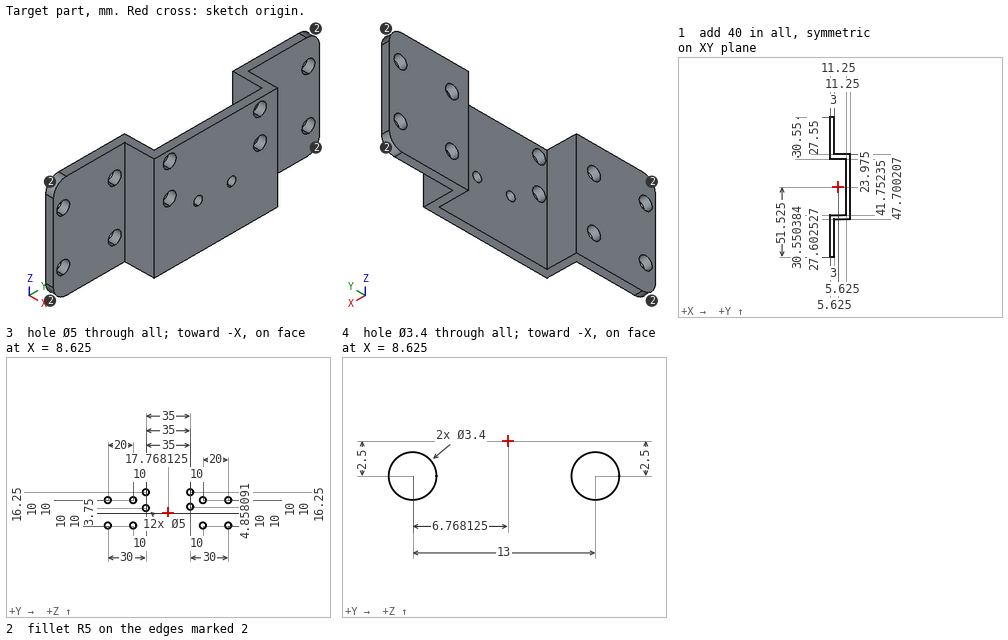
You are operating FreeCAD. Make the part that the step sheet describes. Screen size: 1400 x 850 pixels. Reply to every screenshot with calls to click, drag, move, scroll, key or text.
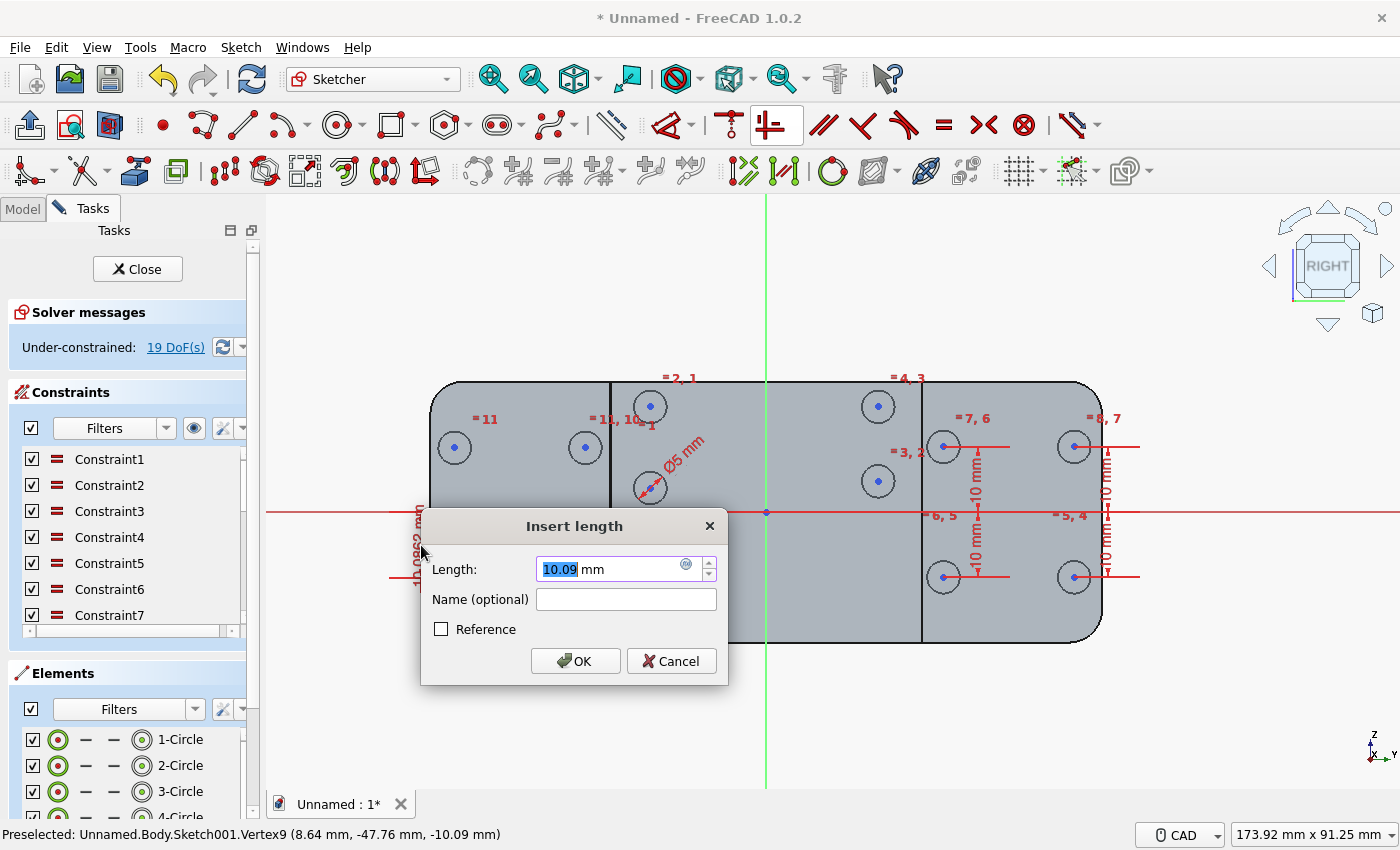
text(10)
key(Return)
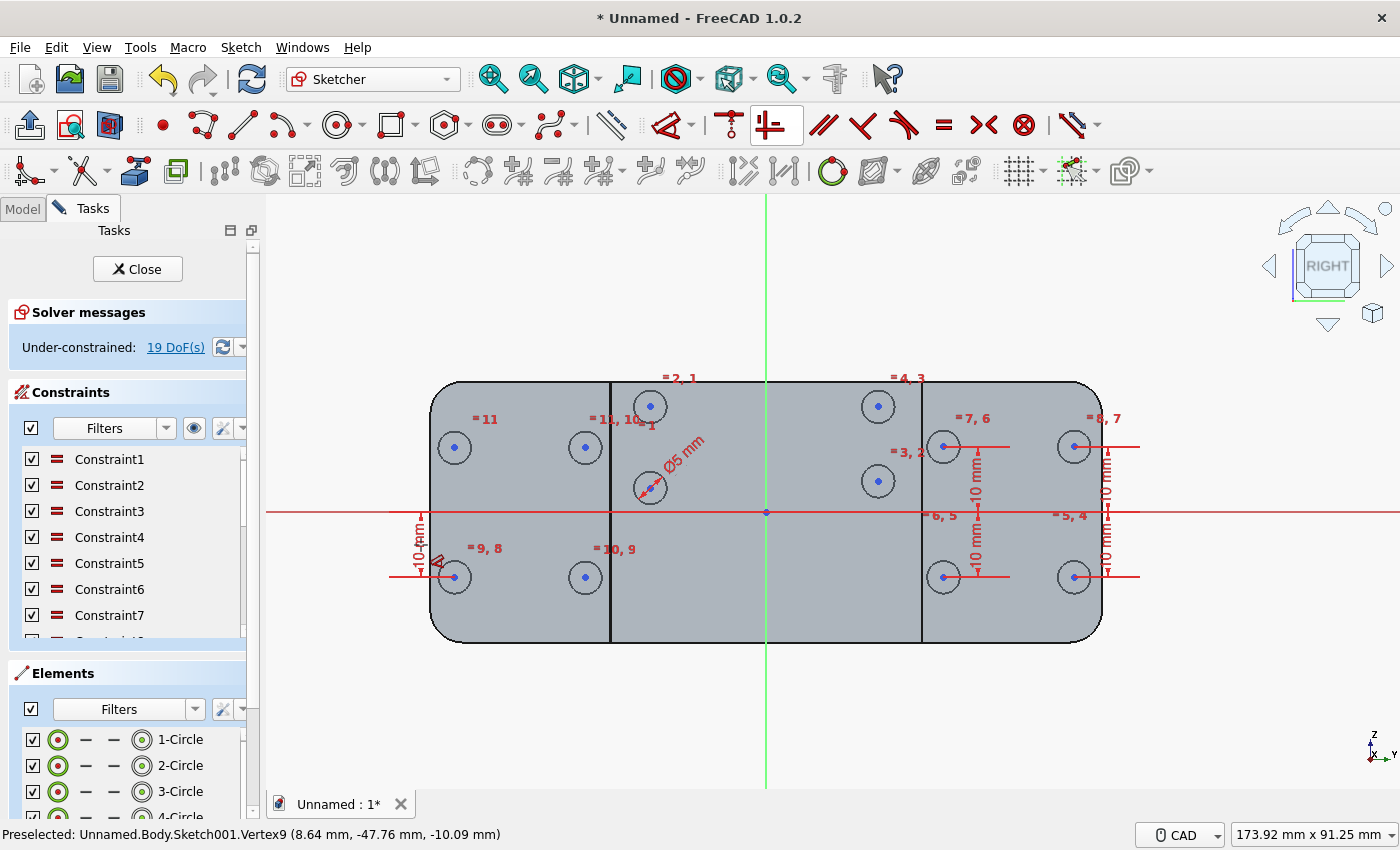
click(585, 578)
click(551, 545)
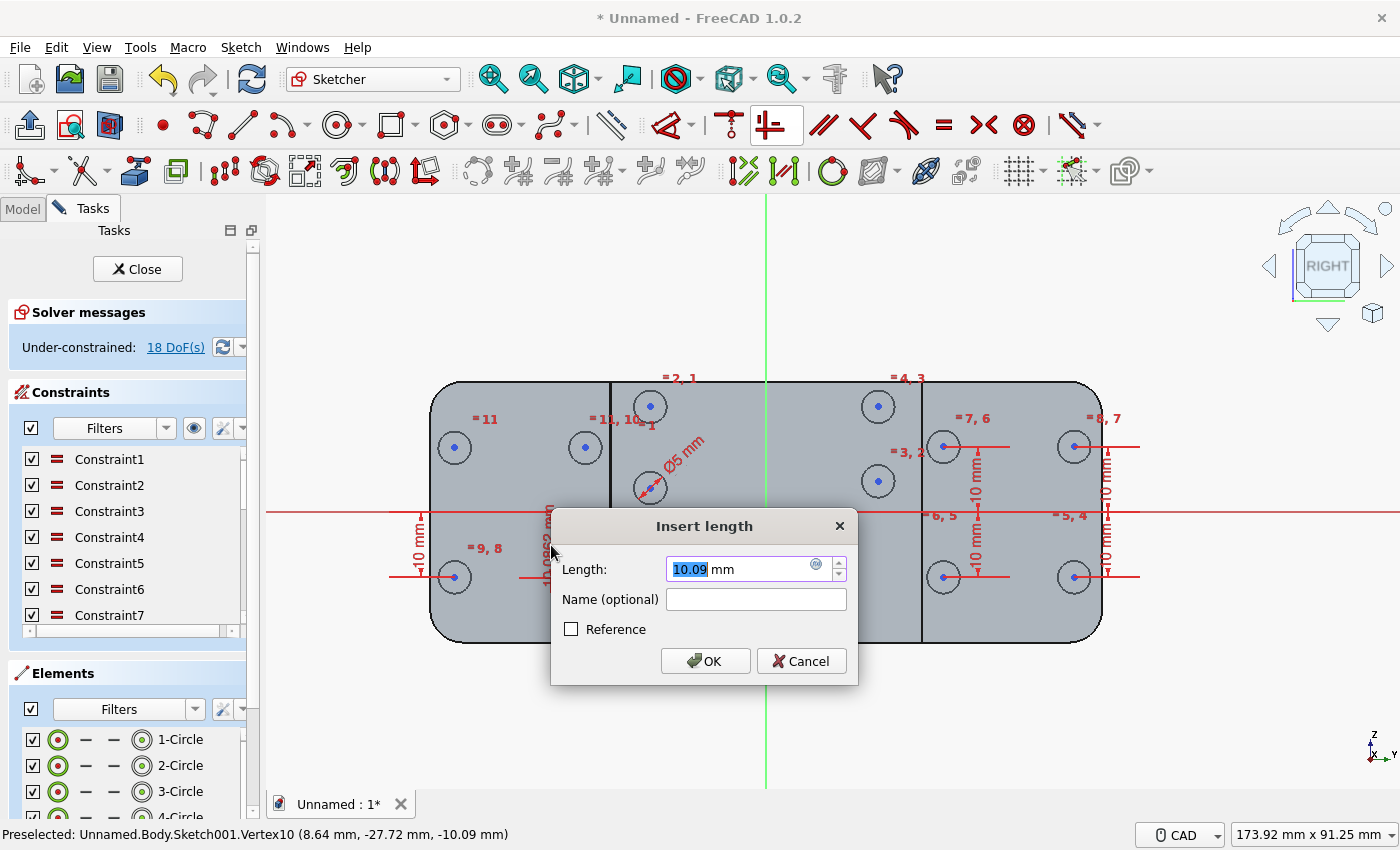
text(10)
key(Return)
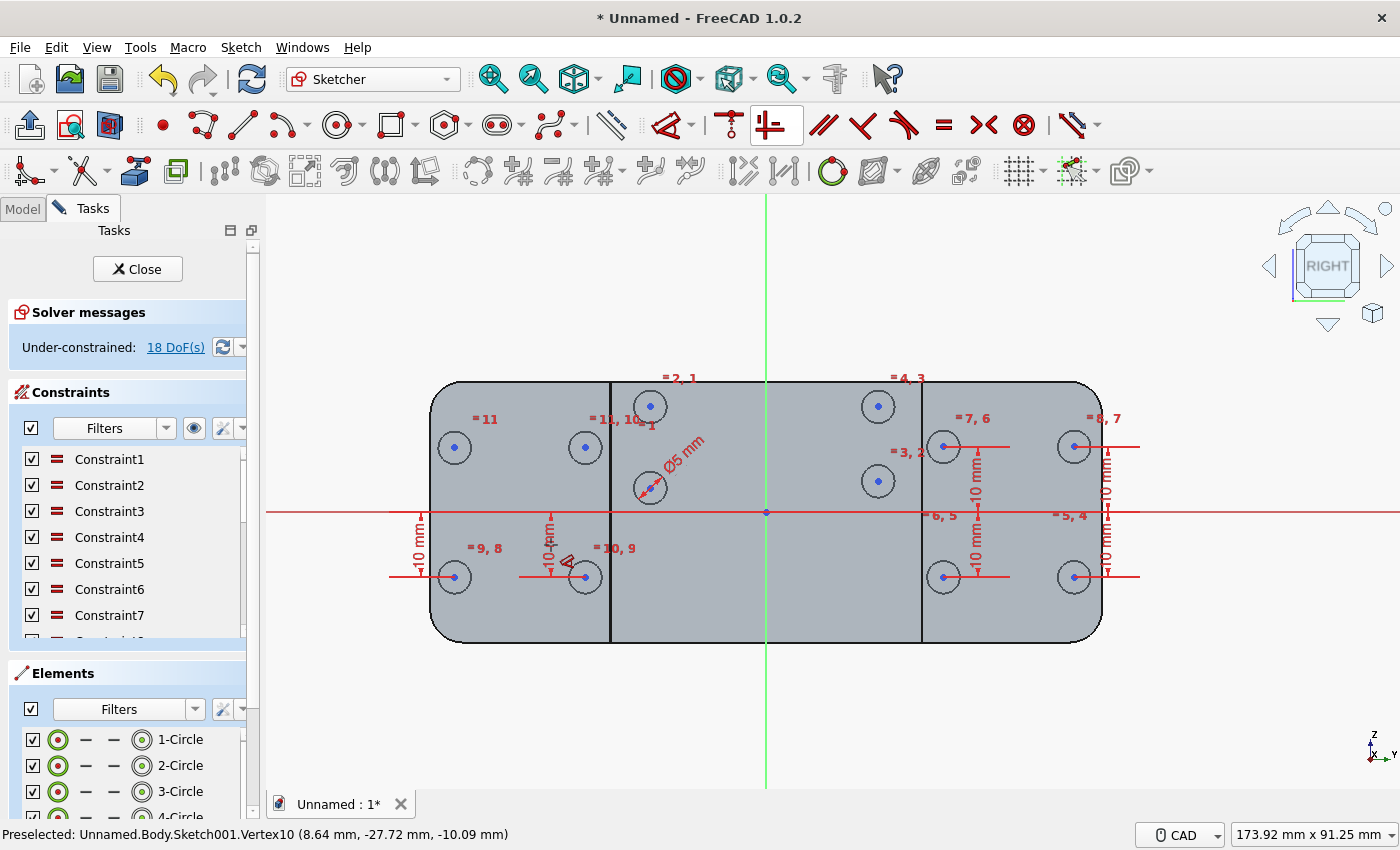
click(585, 448)
click(551, 480)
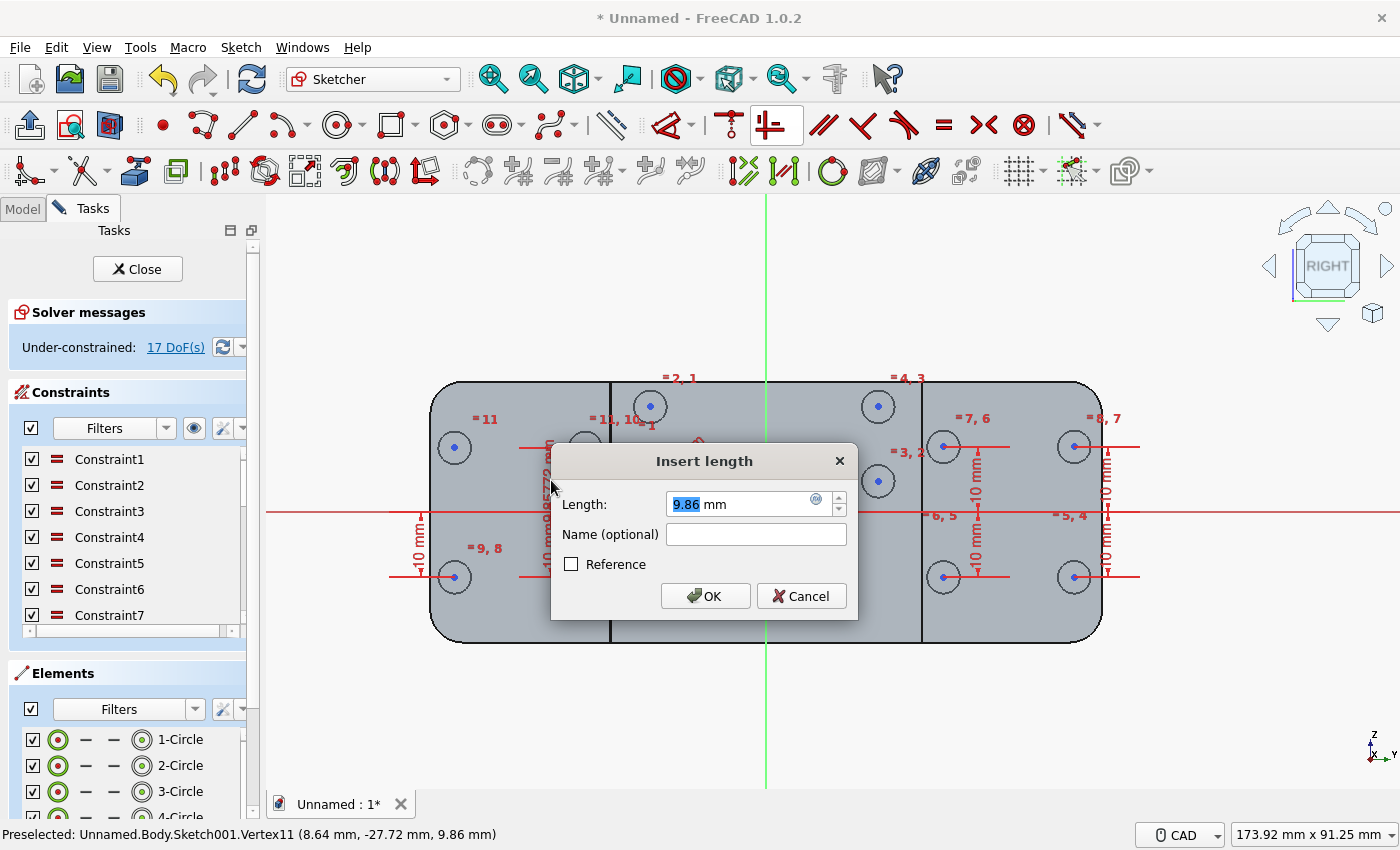
text(10)
key(Return)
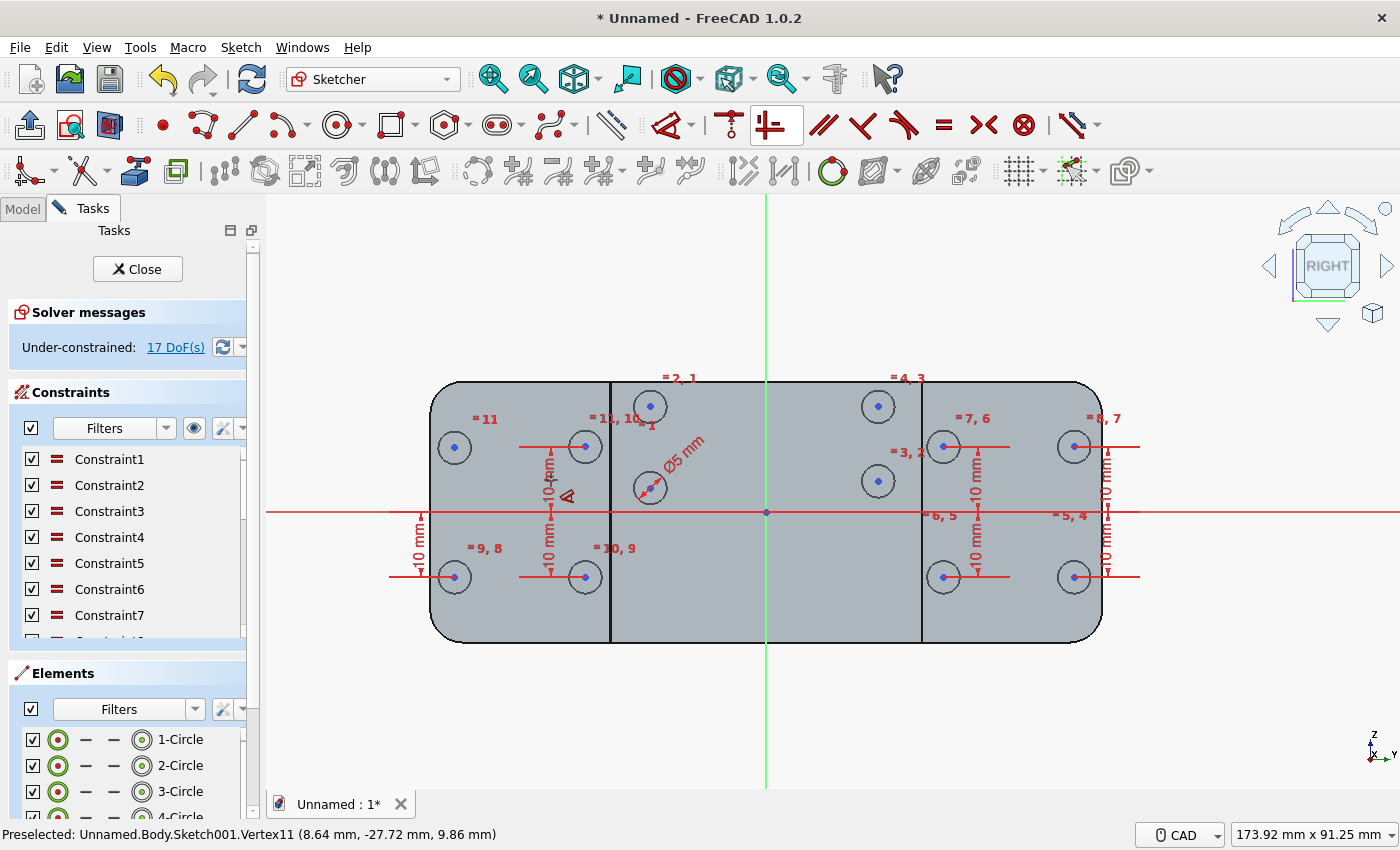
click(455, 448)
click(421, 480)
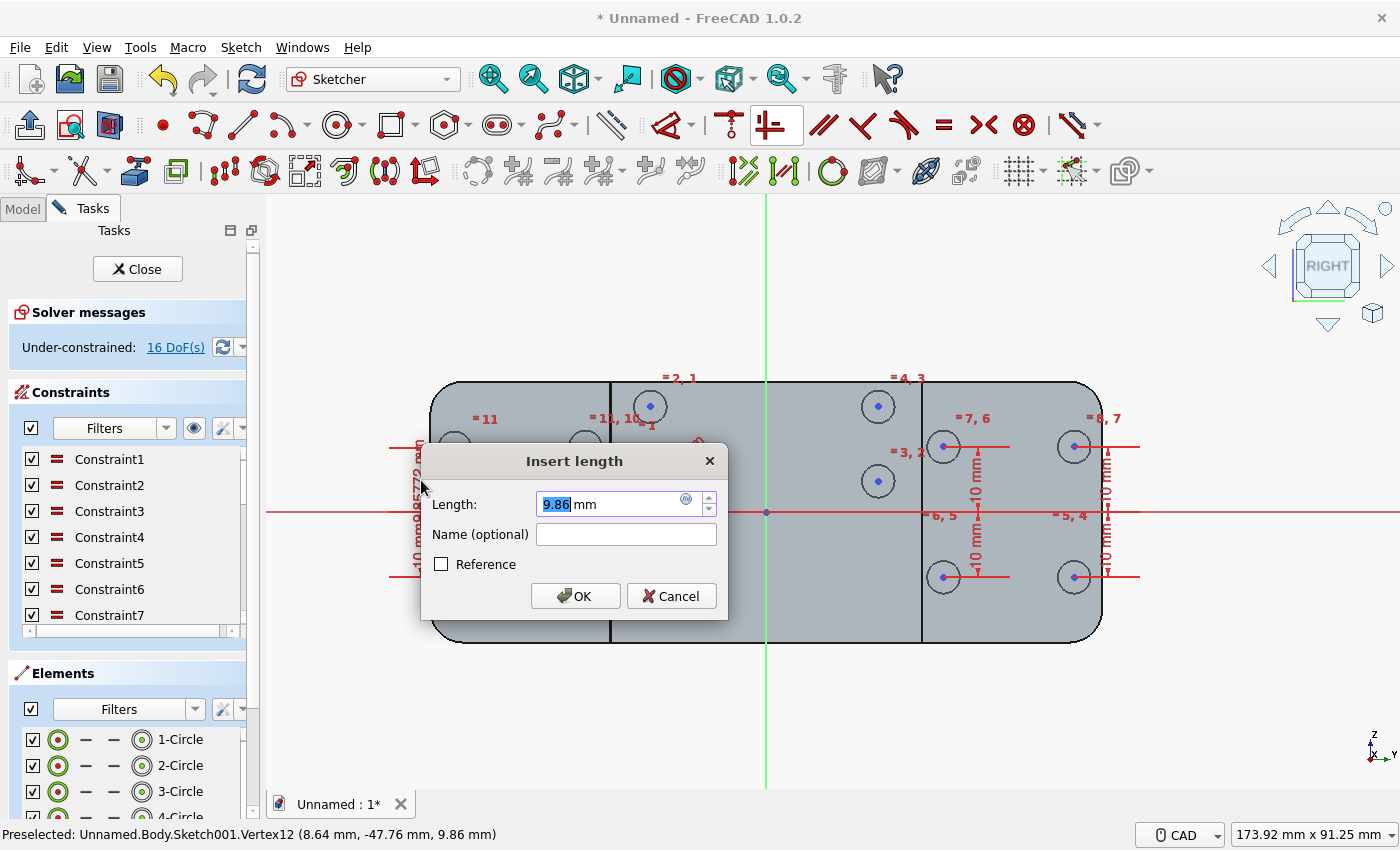
text(10)
key(Return)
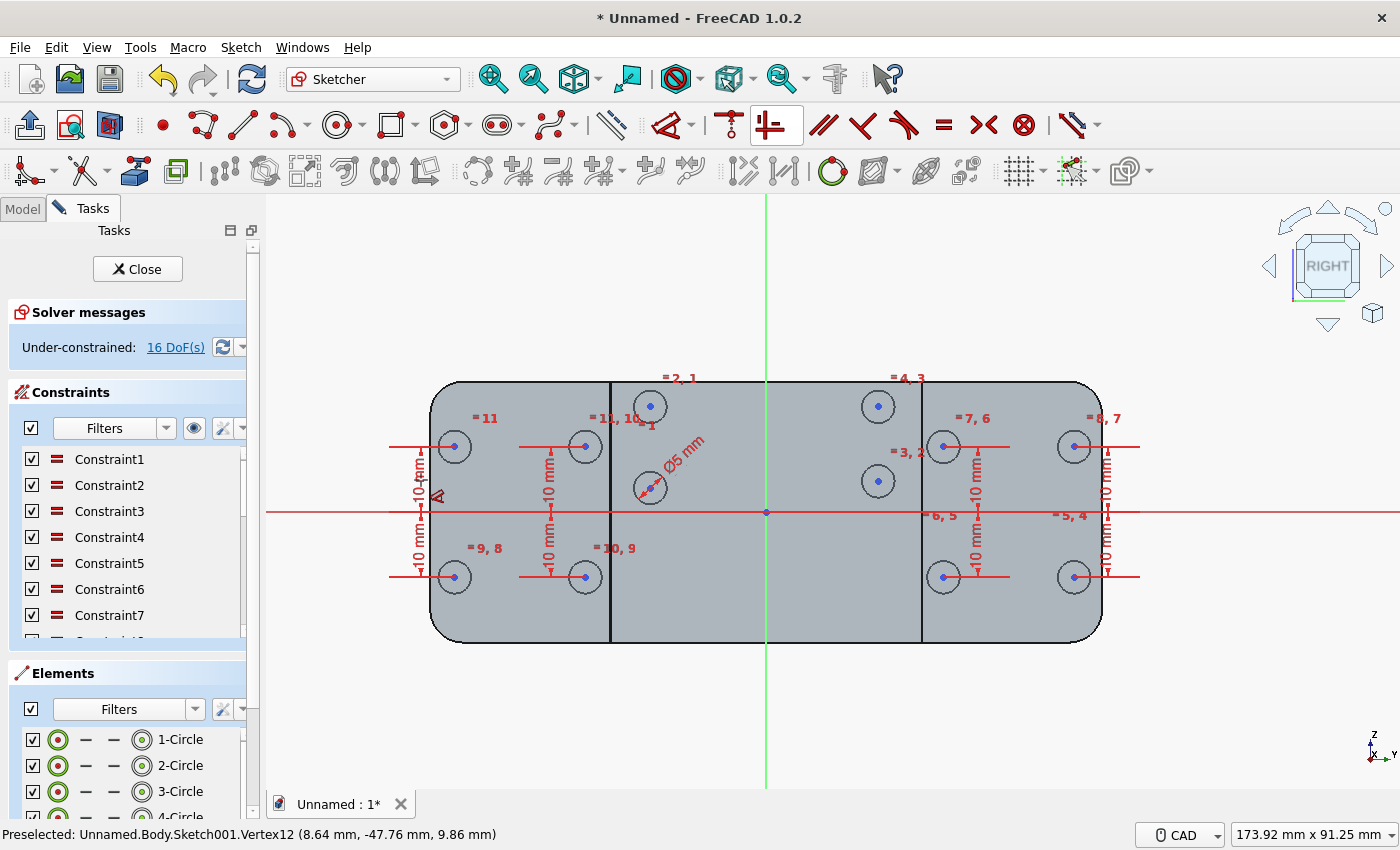
click(650, 488)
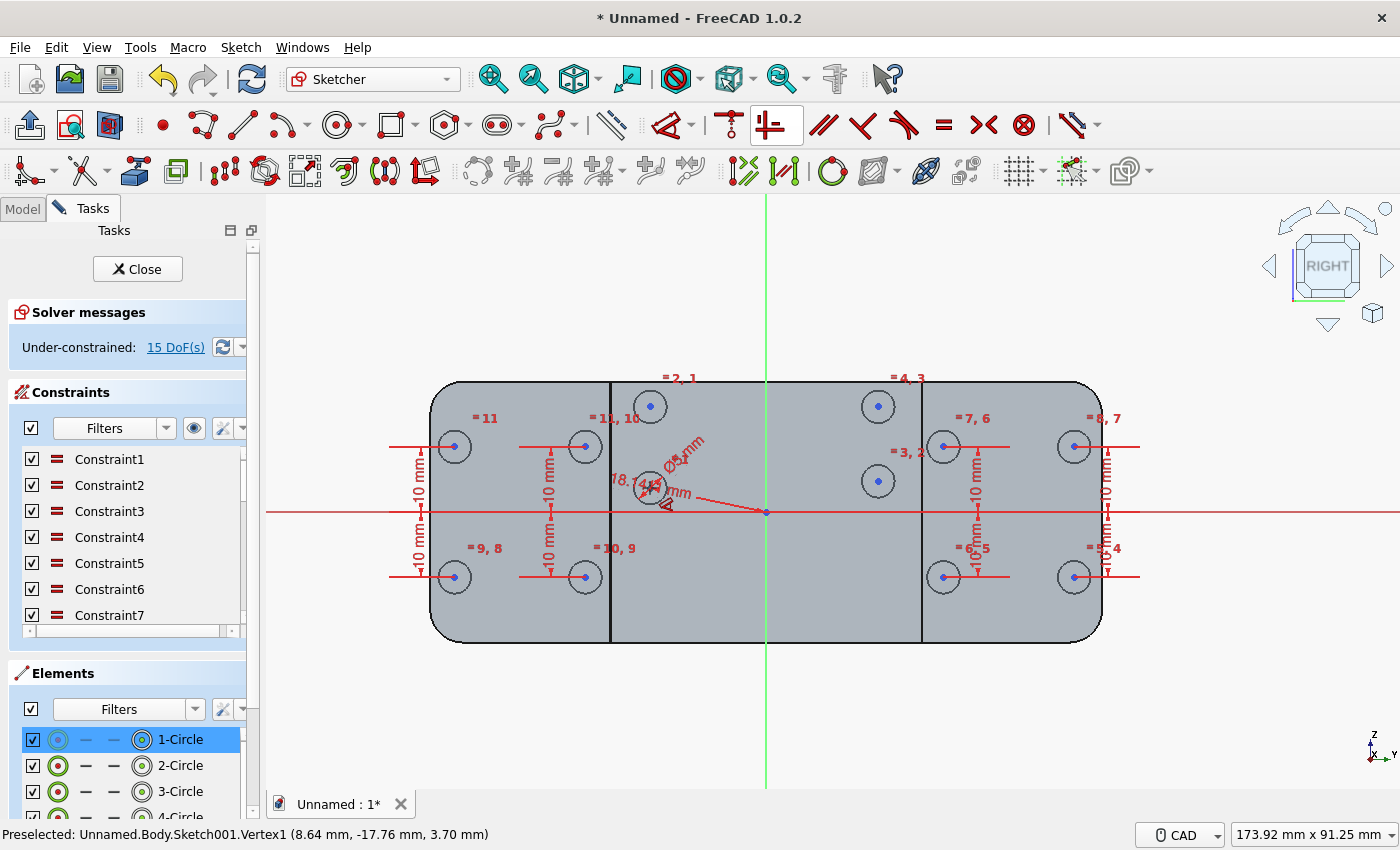
click(878, 481)
click(817, 447)